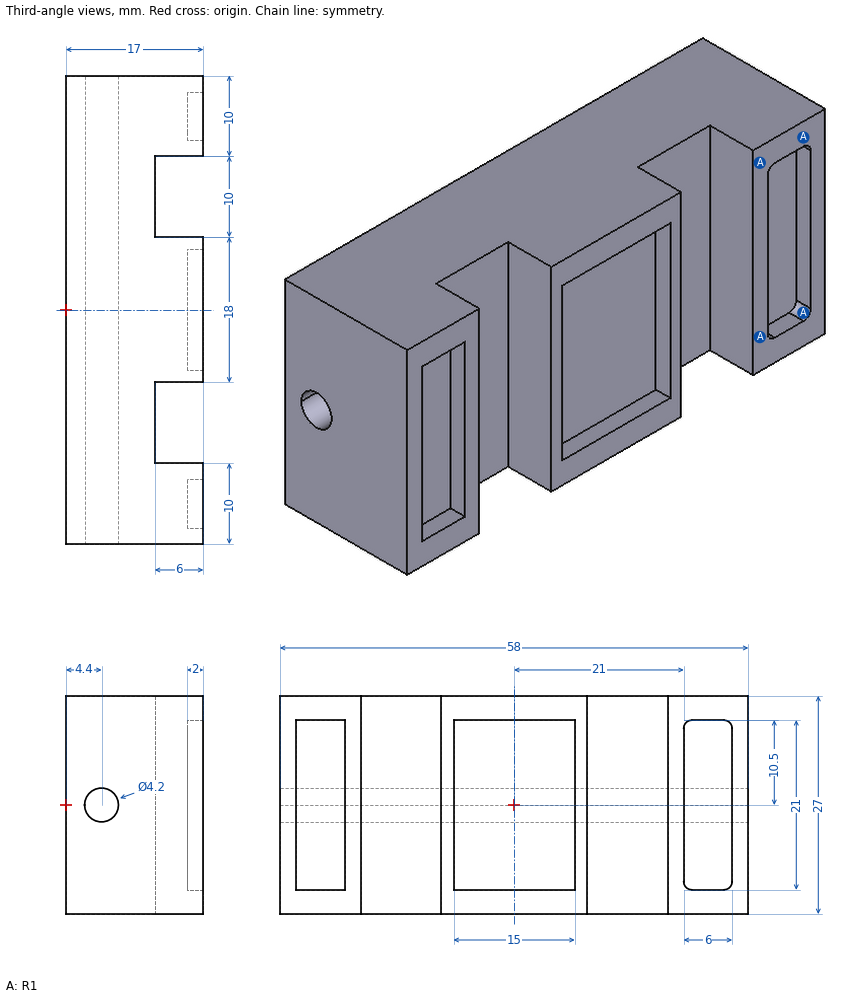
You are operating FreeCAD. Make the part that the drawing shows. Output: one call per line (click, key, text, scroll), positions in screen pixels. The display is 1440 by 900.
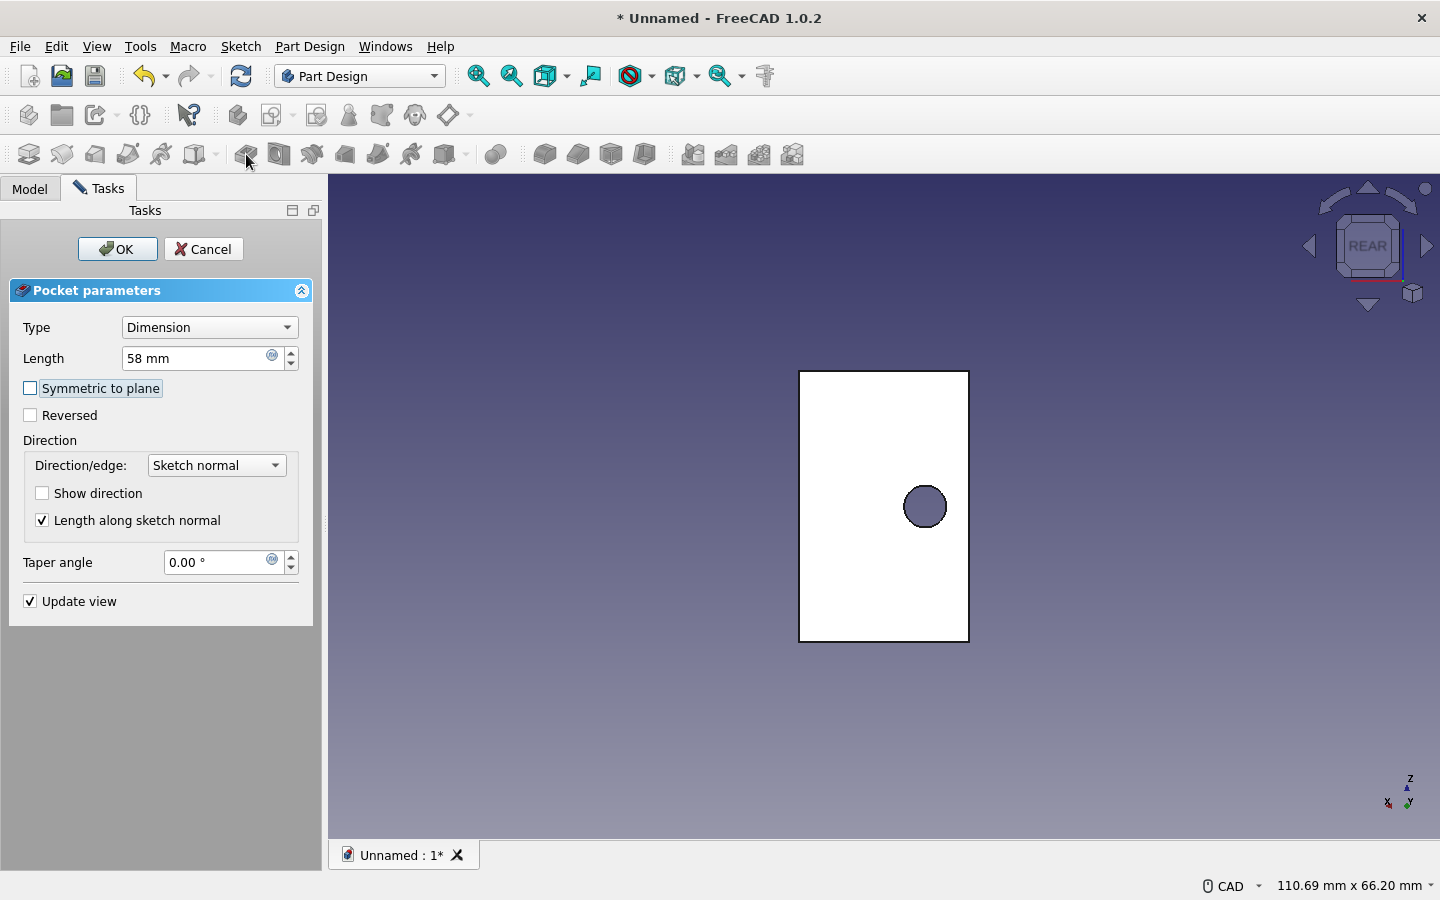
click(118, 249)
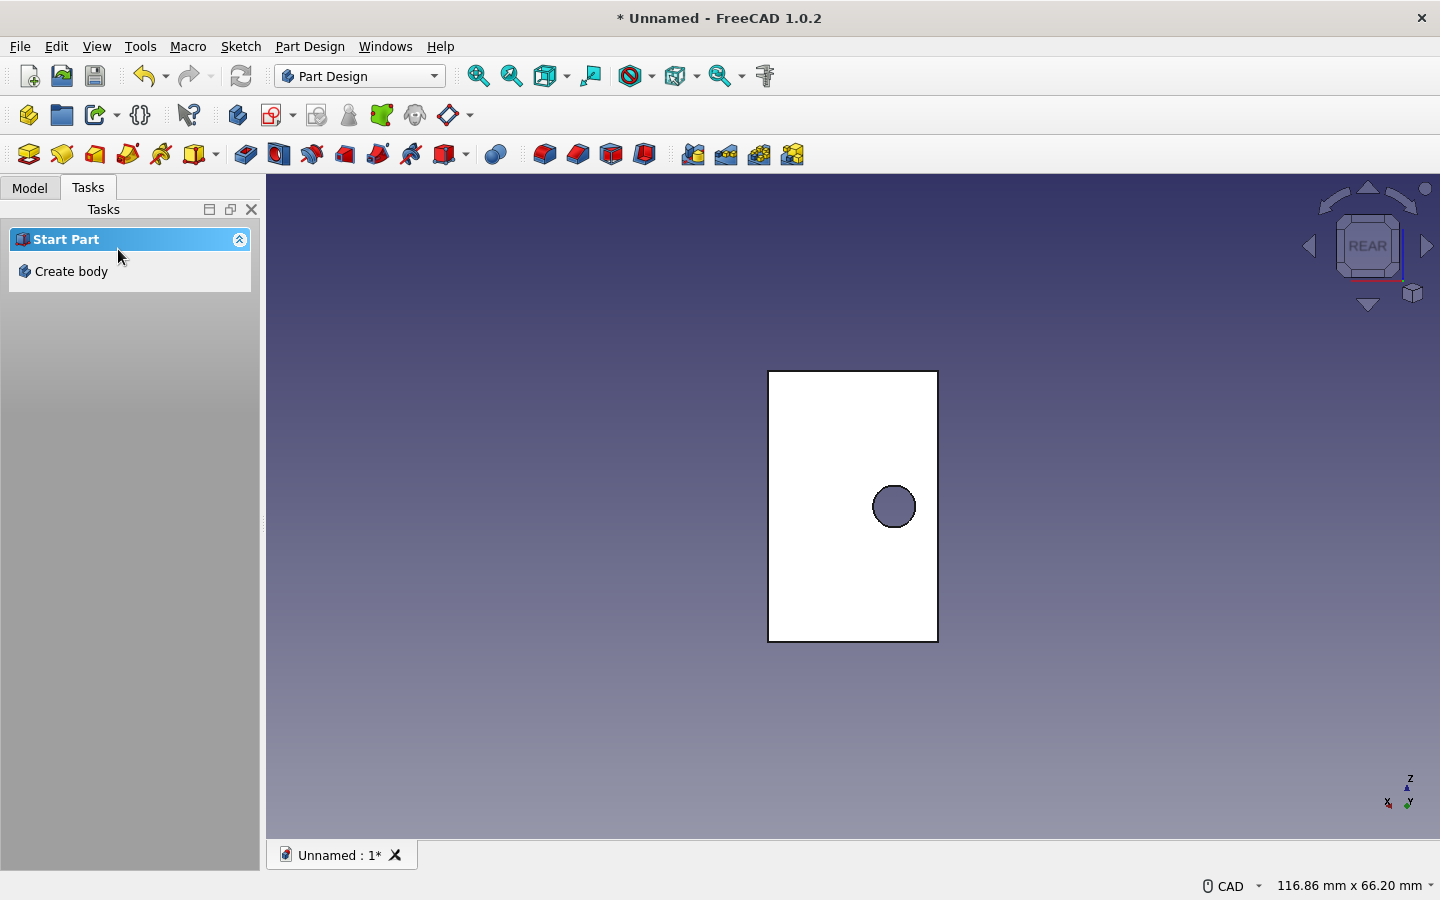
key(v)
key(f)